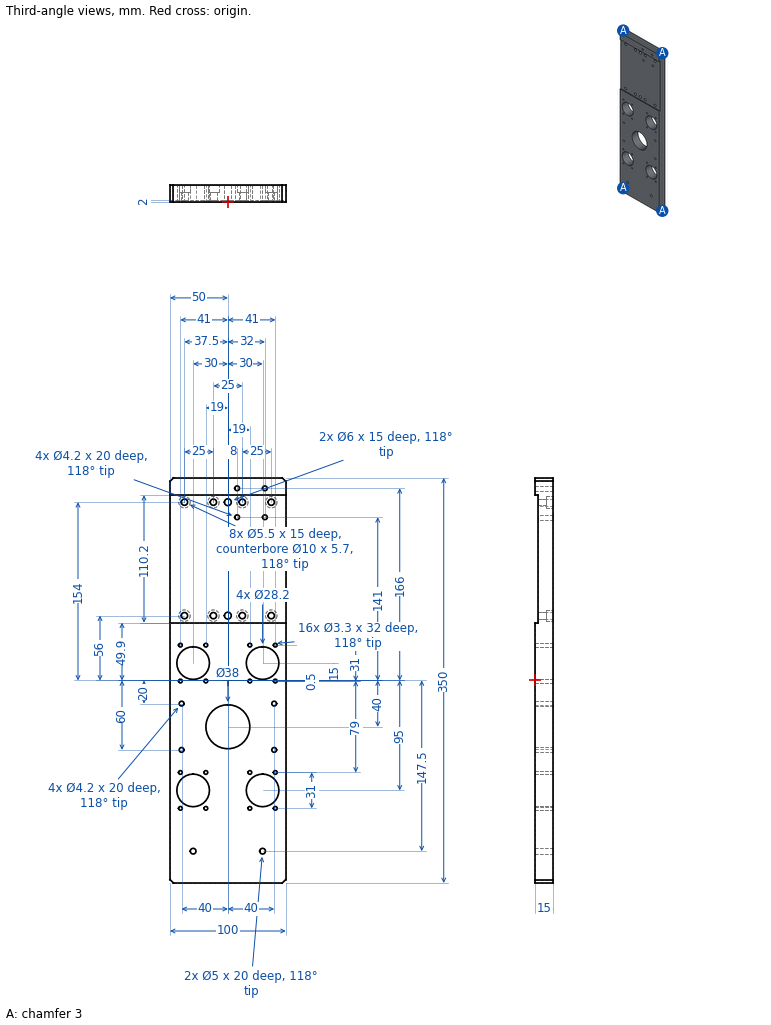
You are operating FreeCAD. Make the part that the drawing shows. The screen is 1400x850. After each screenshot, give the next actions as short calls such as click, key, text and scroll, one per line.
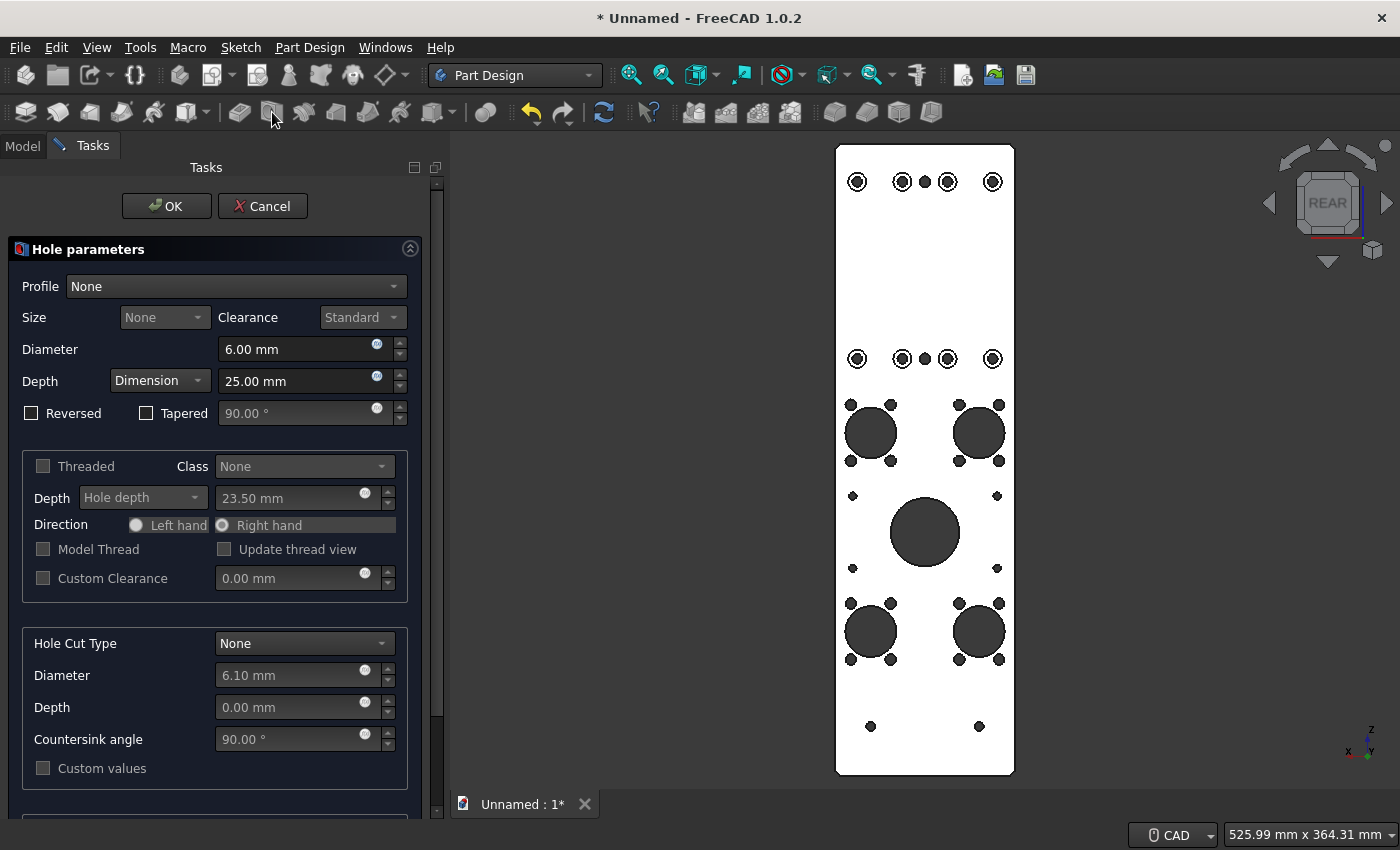
triple_click(305, 349)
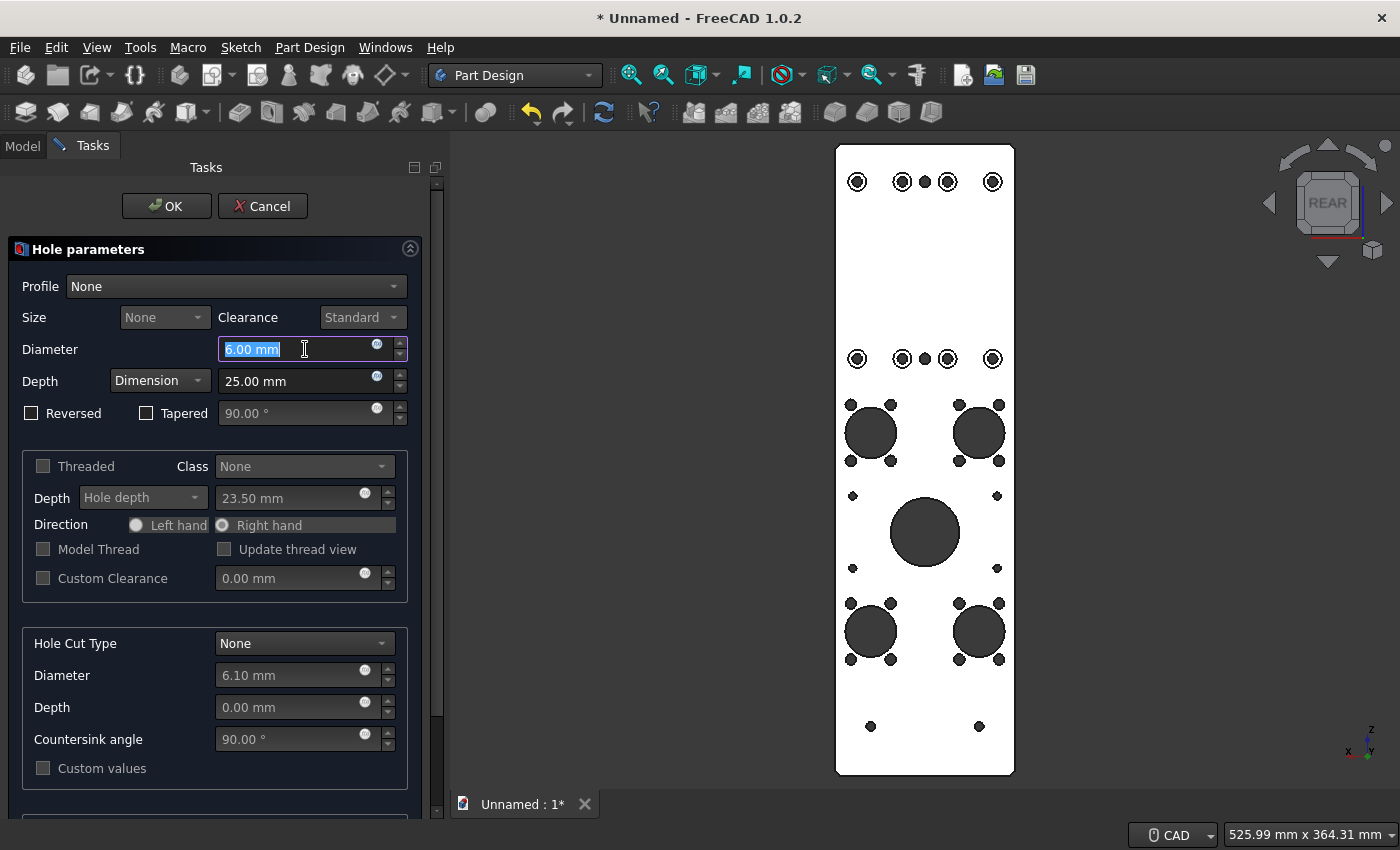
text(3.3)
key(Tab)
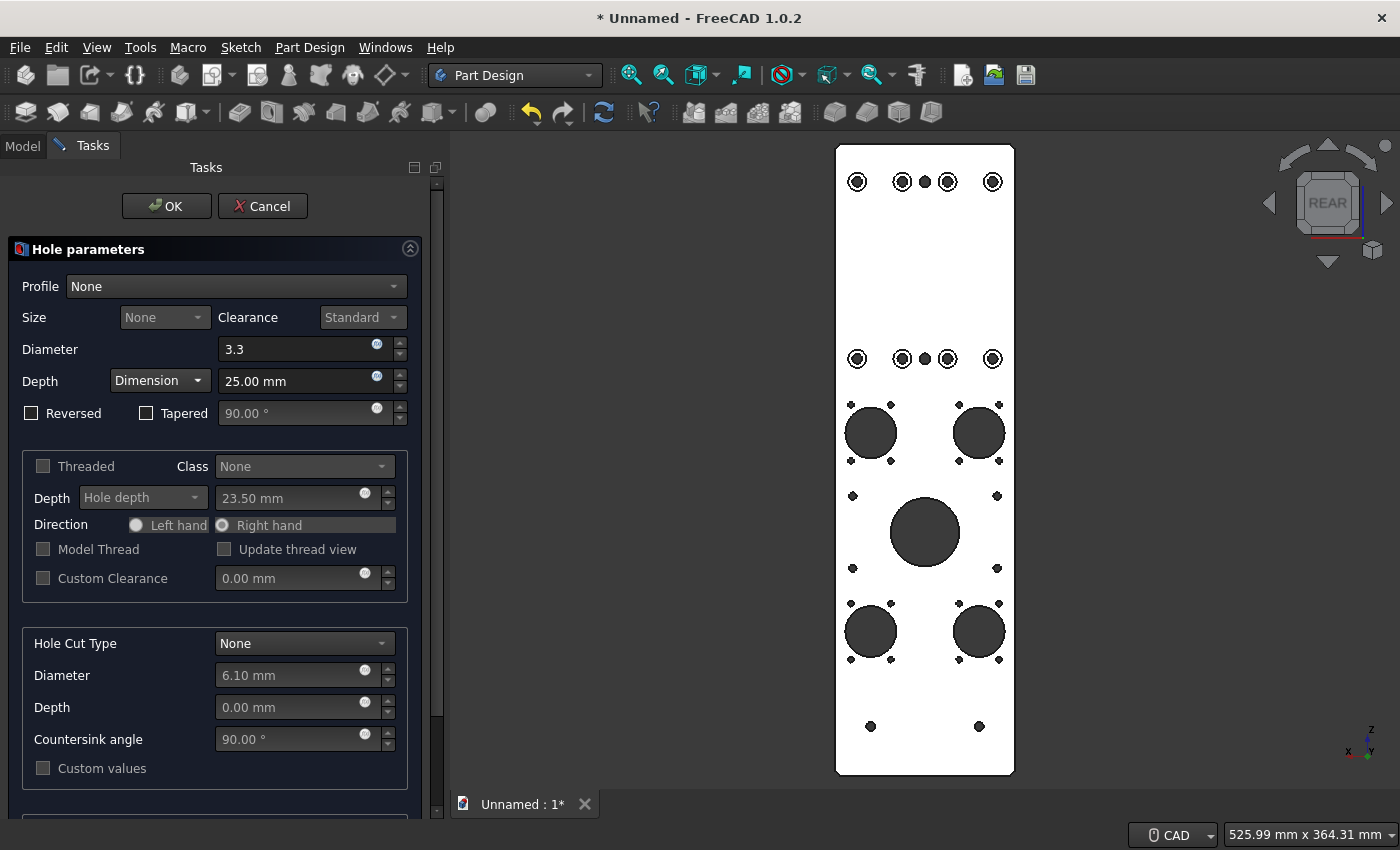
triple_click(305, 381)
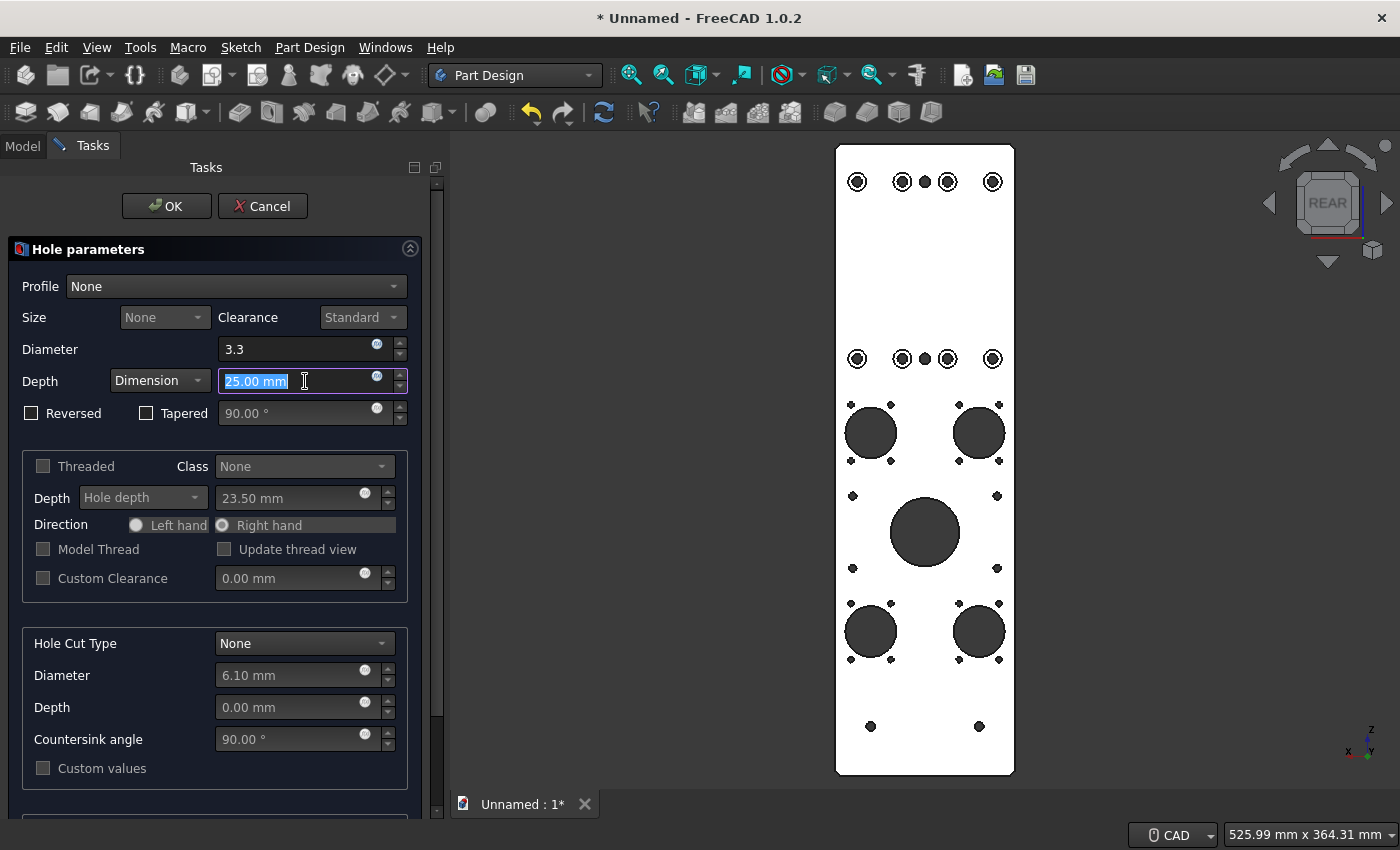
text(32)
key(Tab)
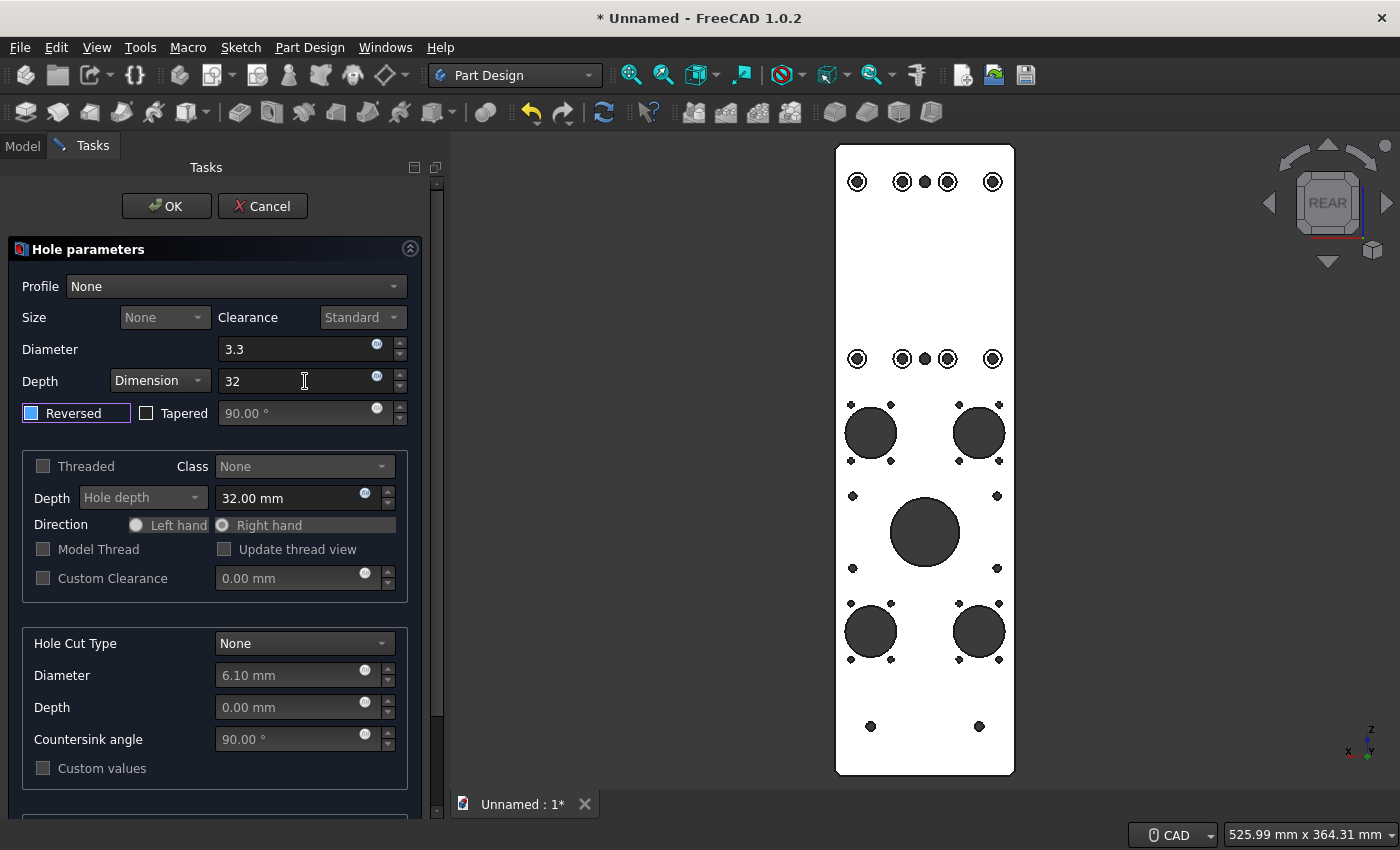
click(167, 206)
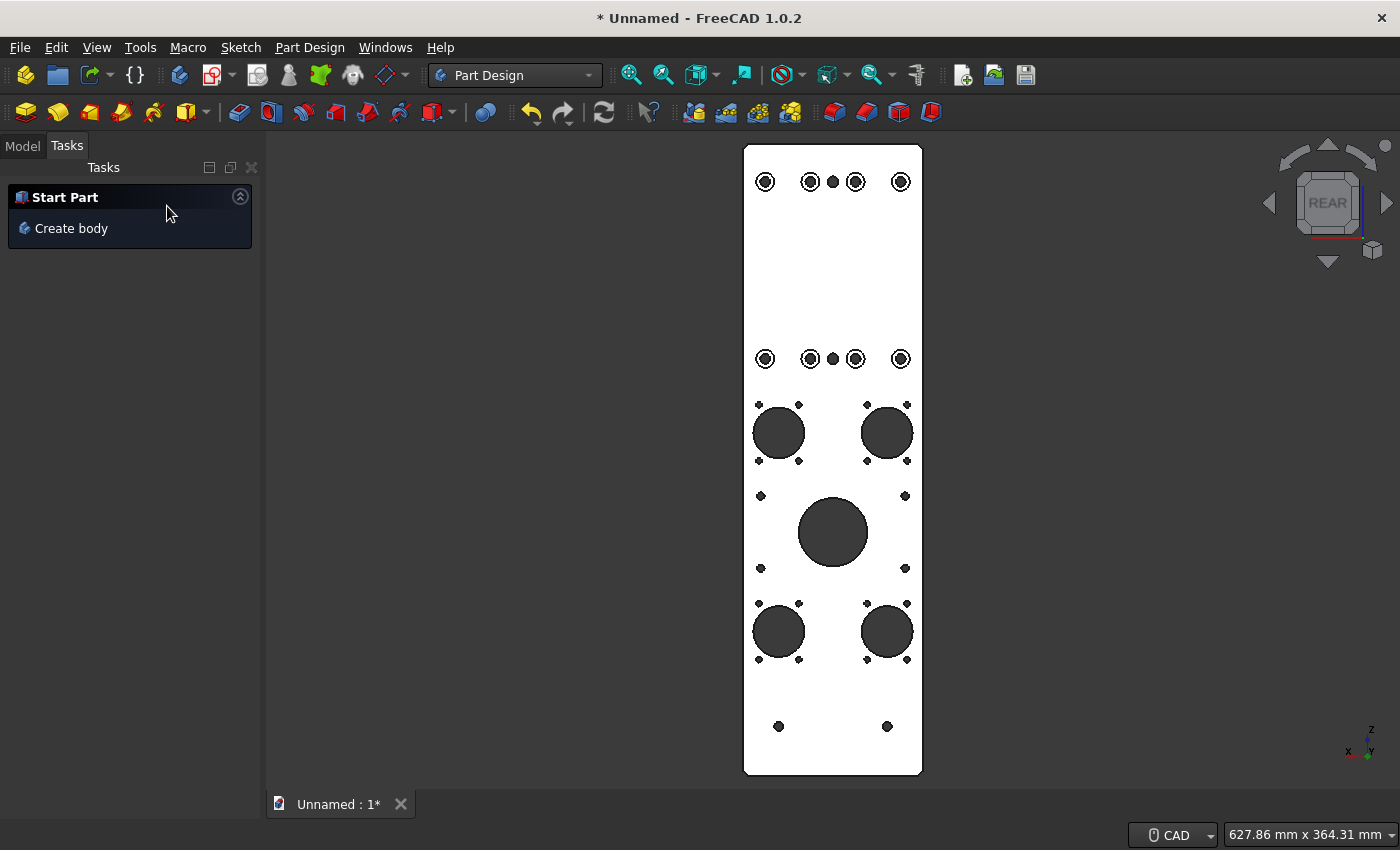
click(833, 278)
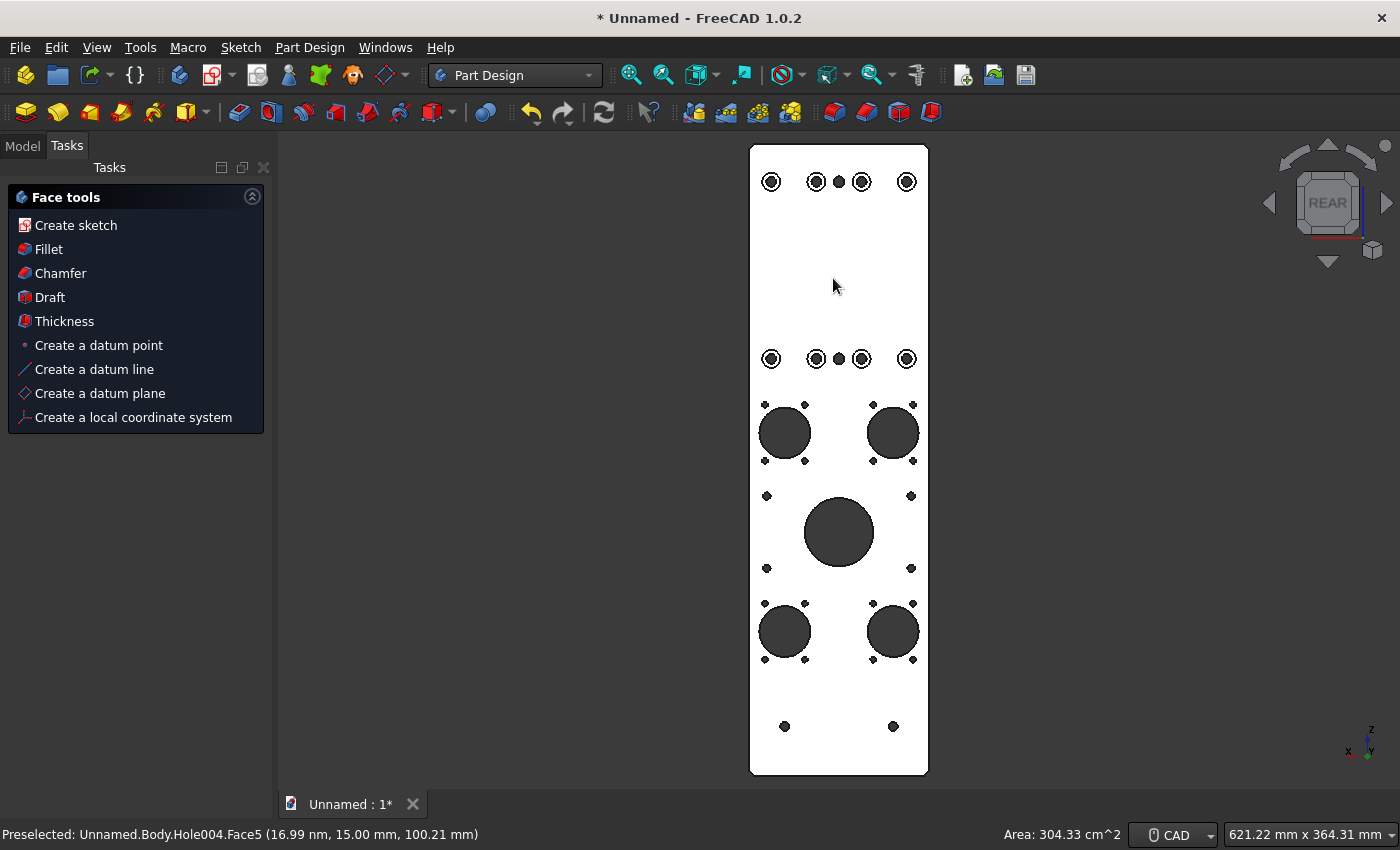
click(212, 76)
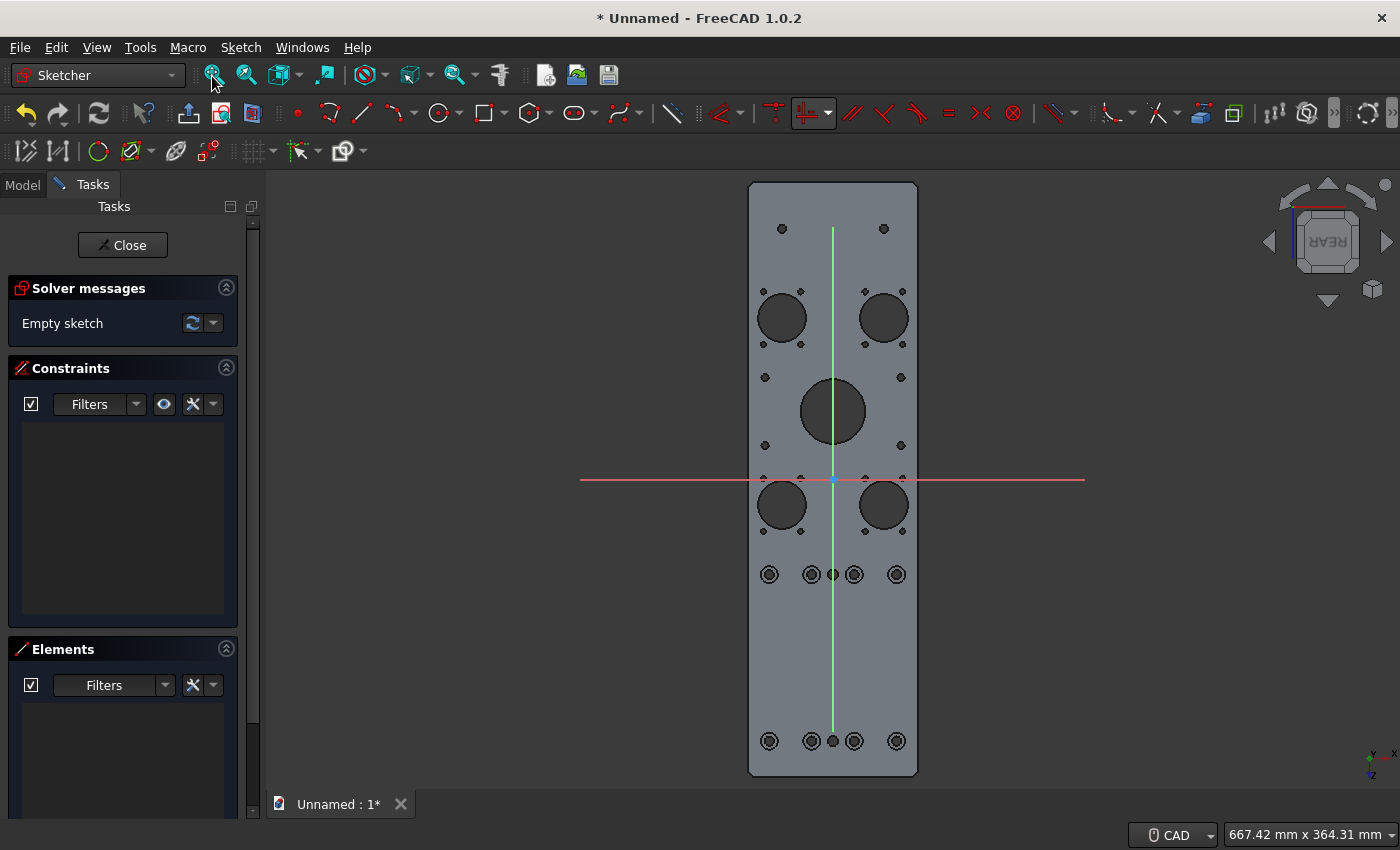
scroll(764, 480, down, 5)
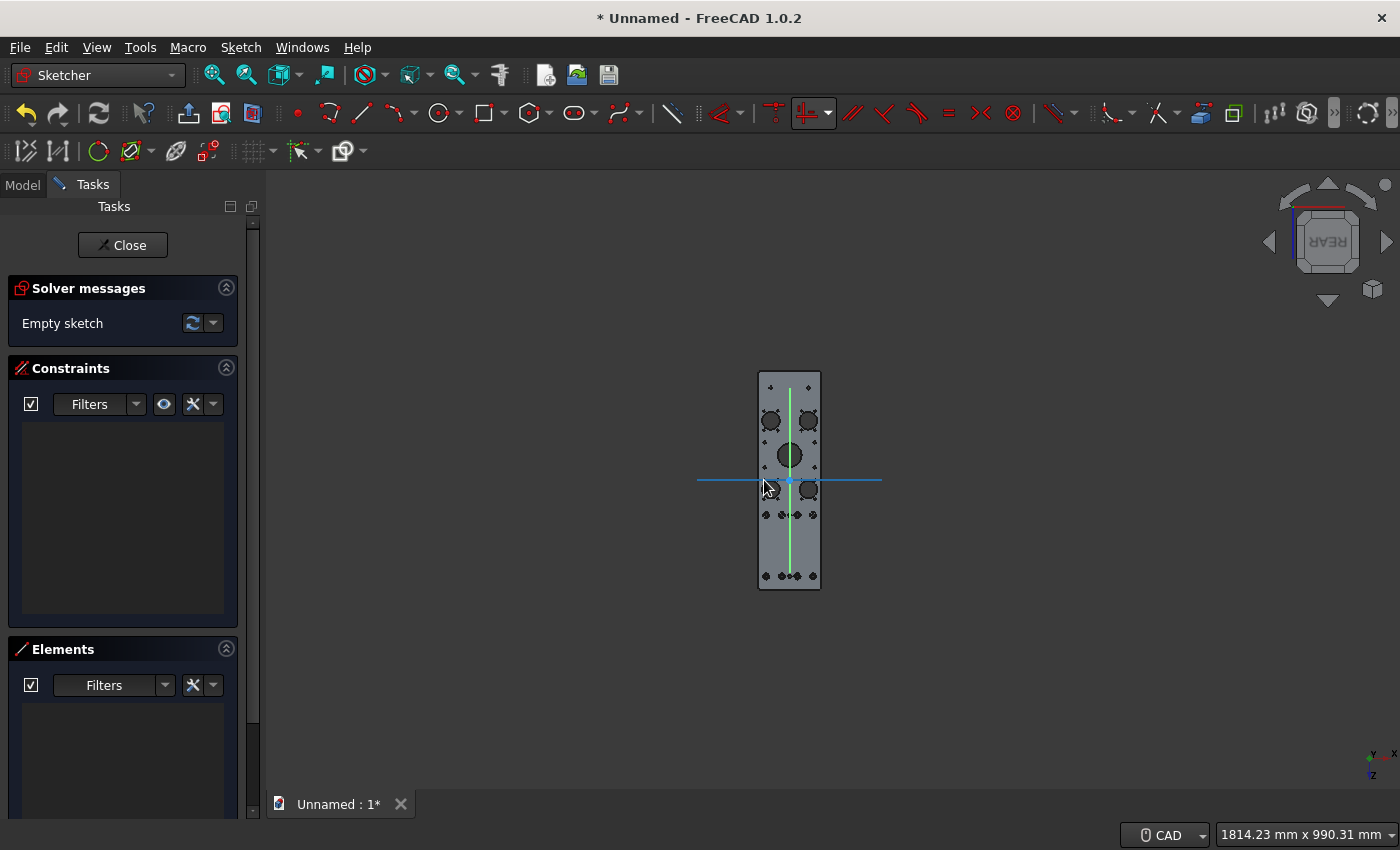
scroll(804, 581, up, 15)